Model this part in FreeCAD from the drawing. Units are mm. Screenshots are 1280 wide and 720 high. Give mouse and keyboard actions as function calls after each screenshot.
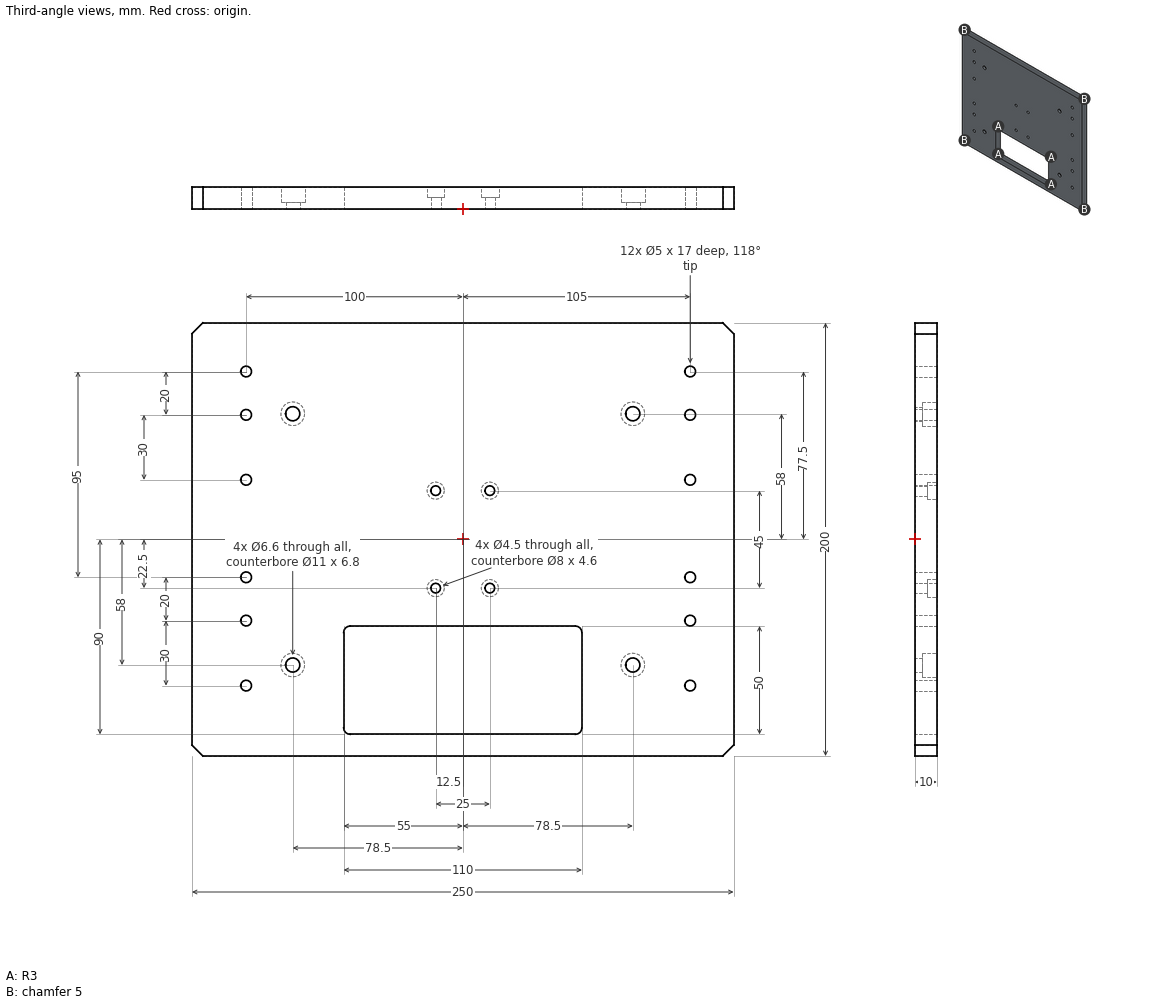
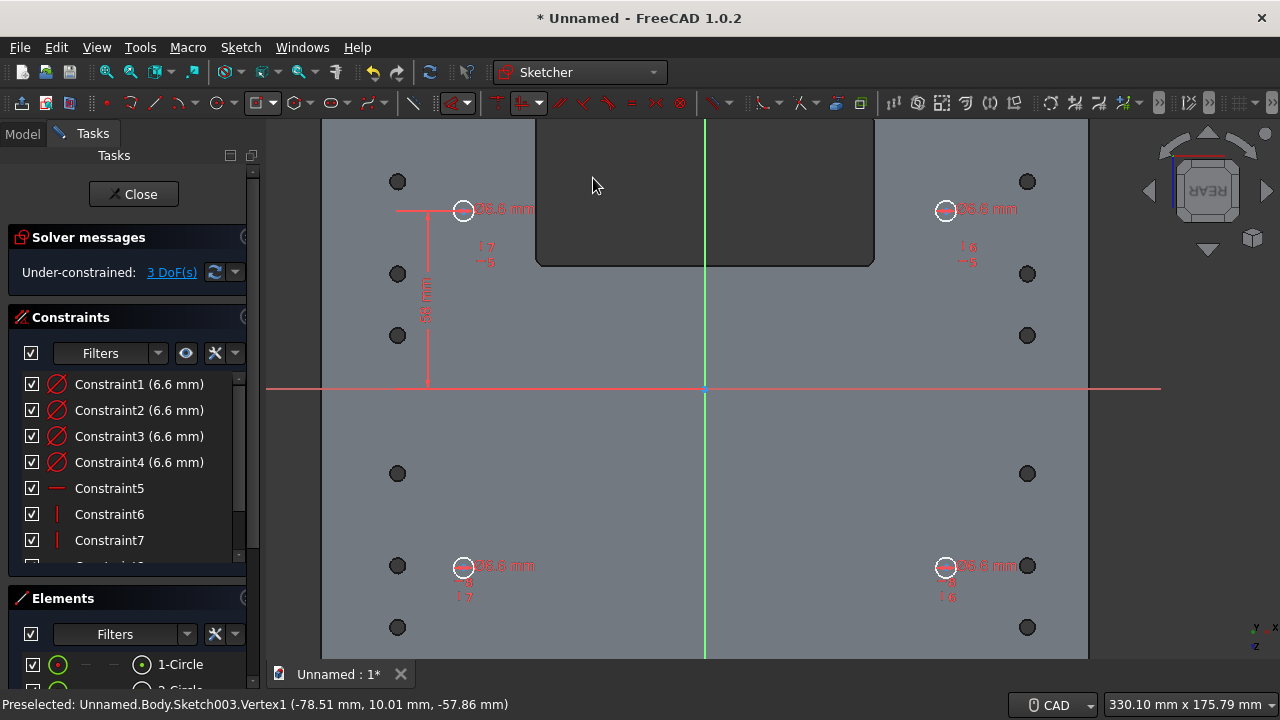
click(946, 568)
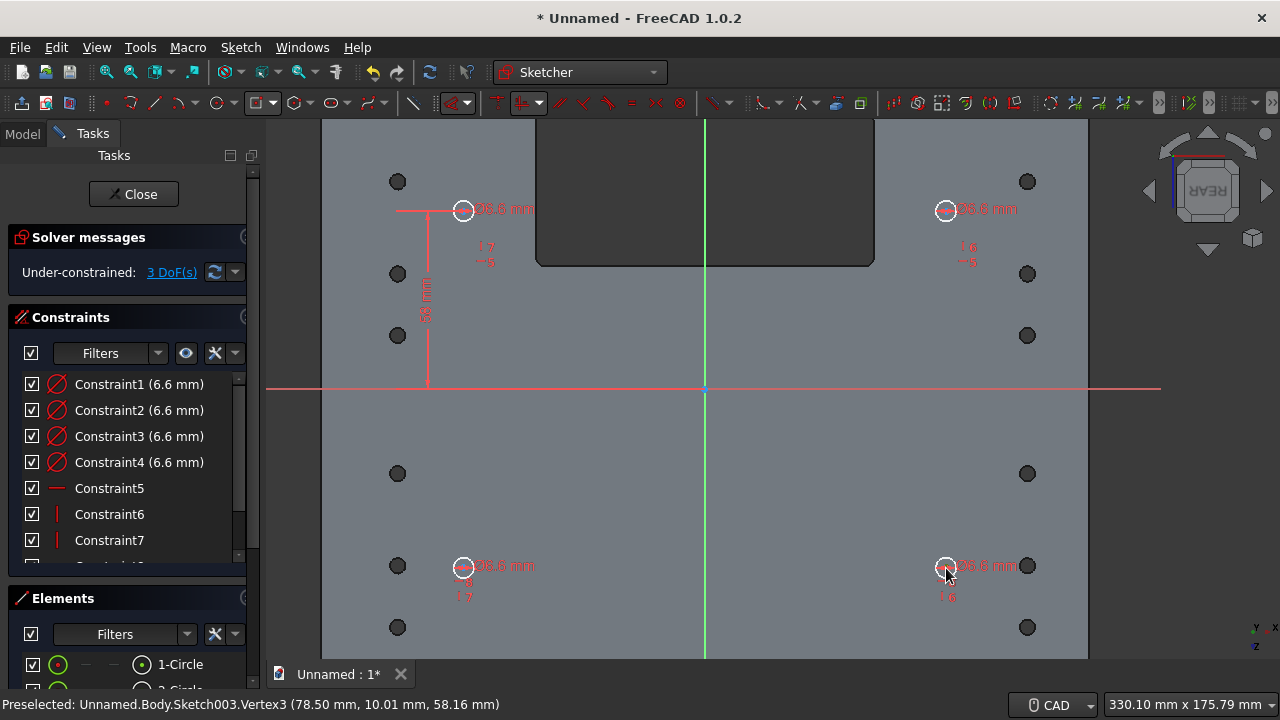
key(i)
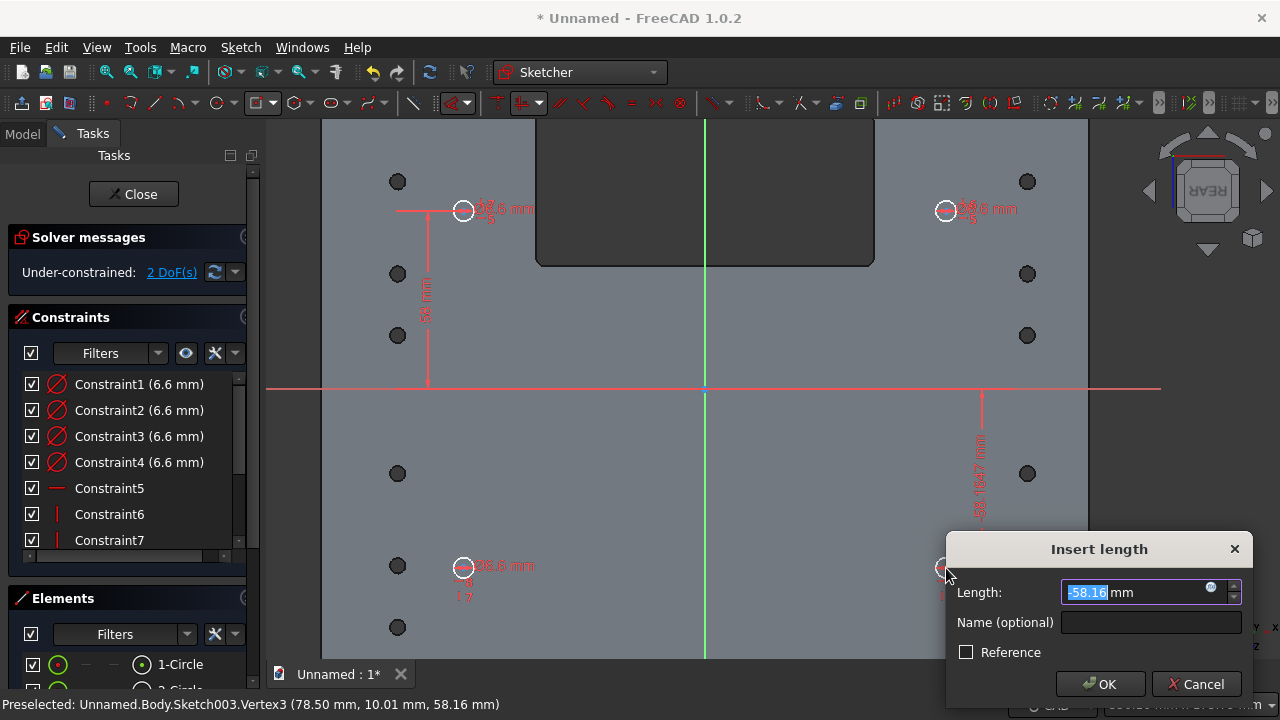
text(-58)
key(Return)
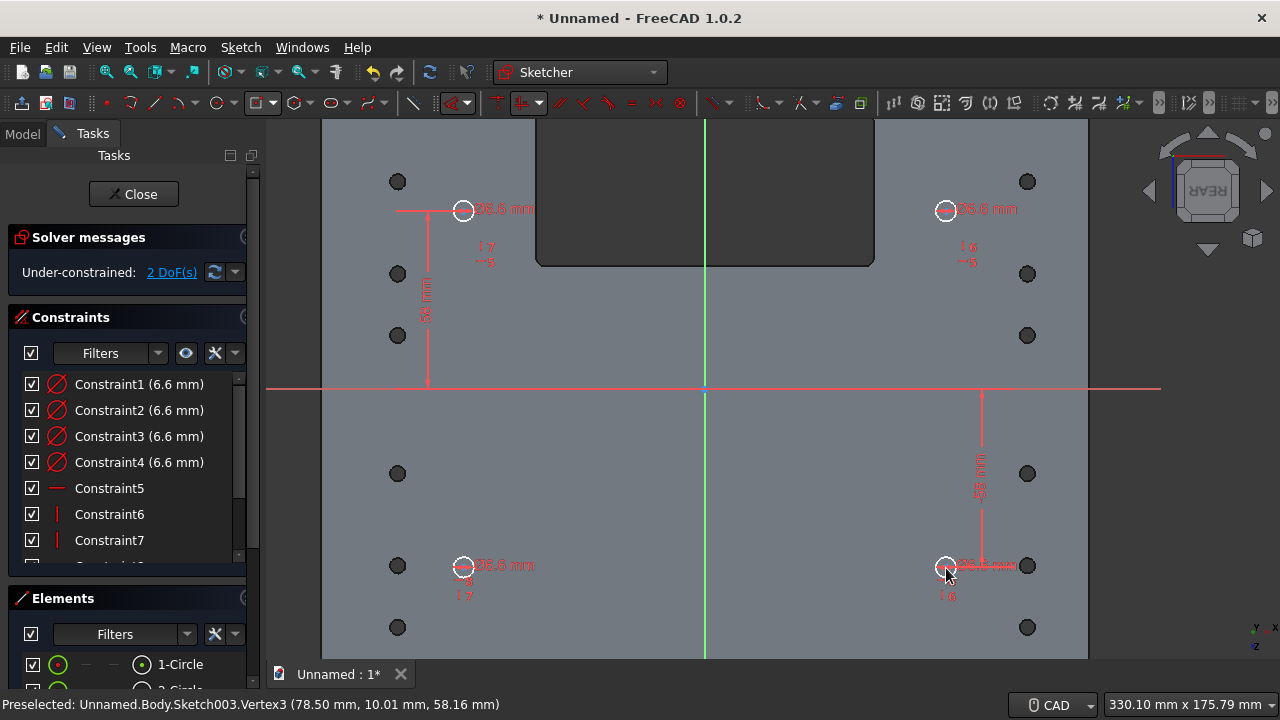
click(464, 211)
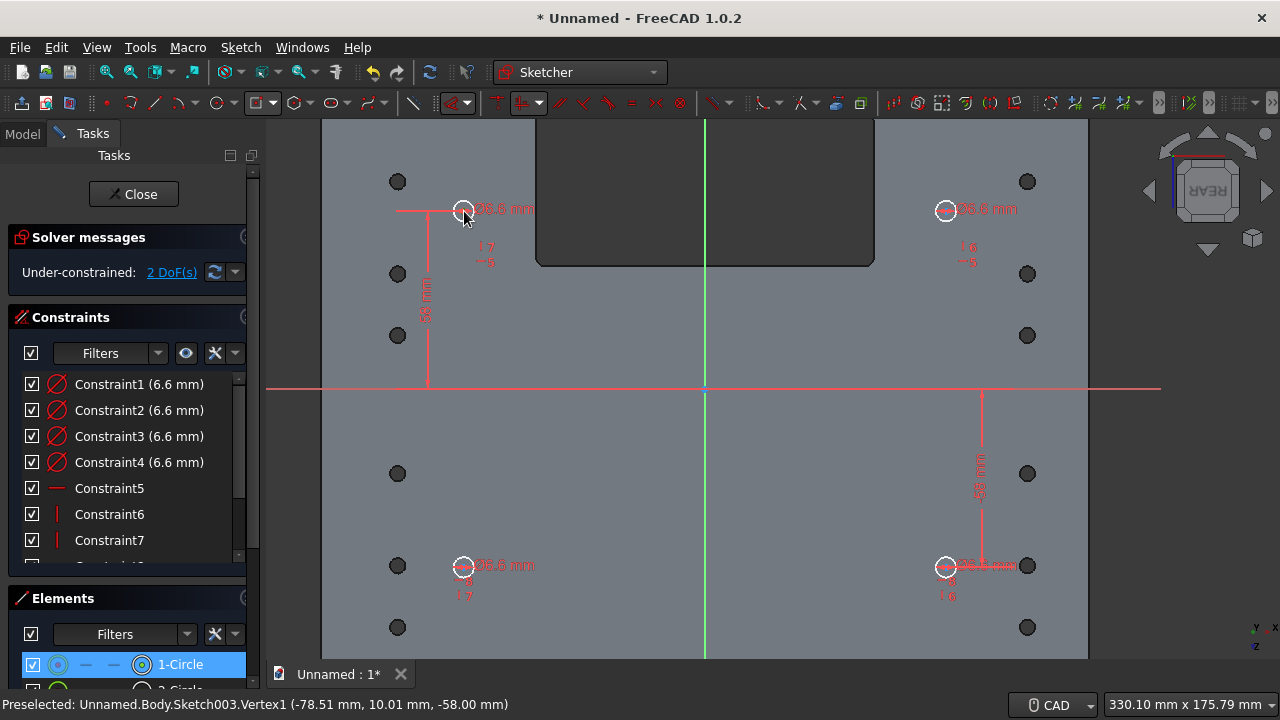
click(470, 104)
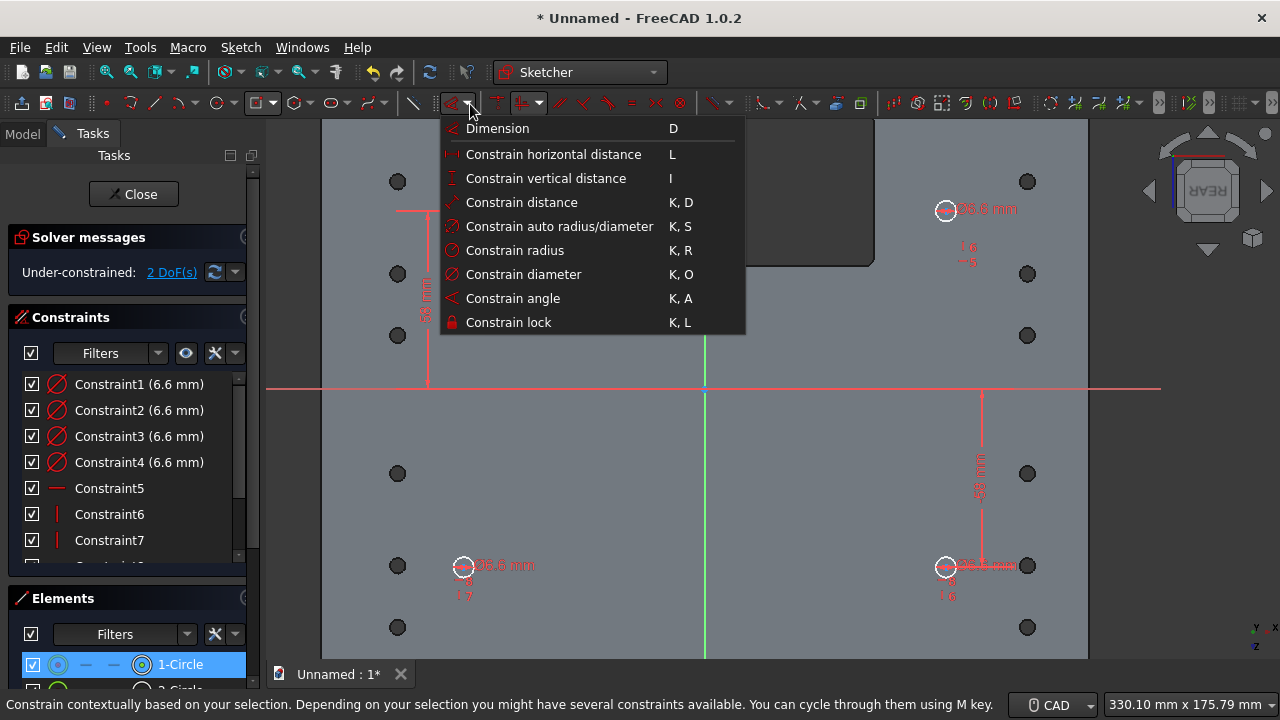
click(593, 154)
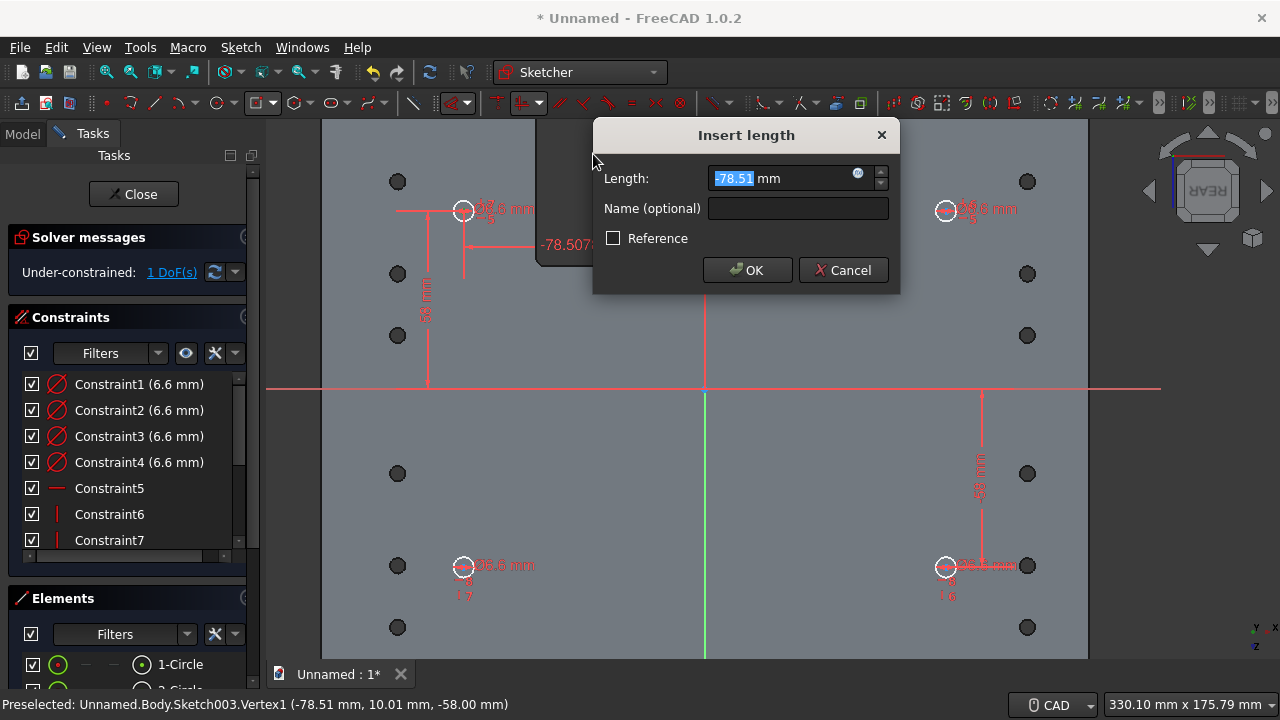
text(-78.5)
key(Return)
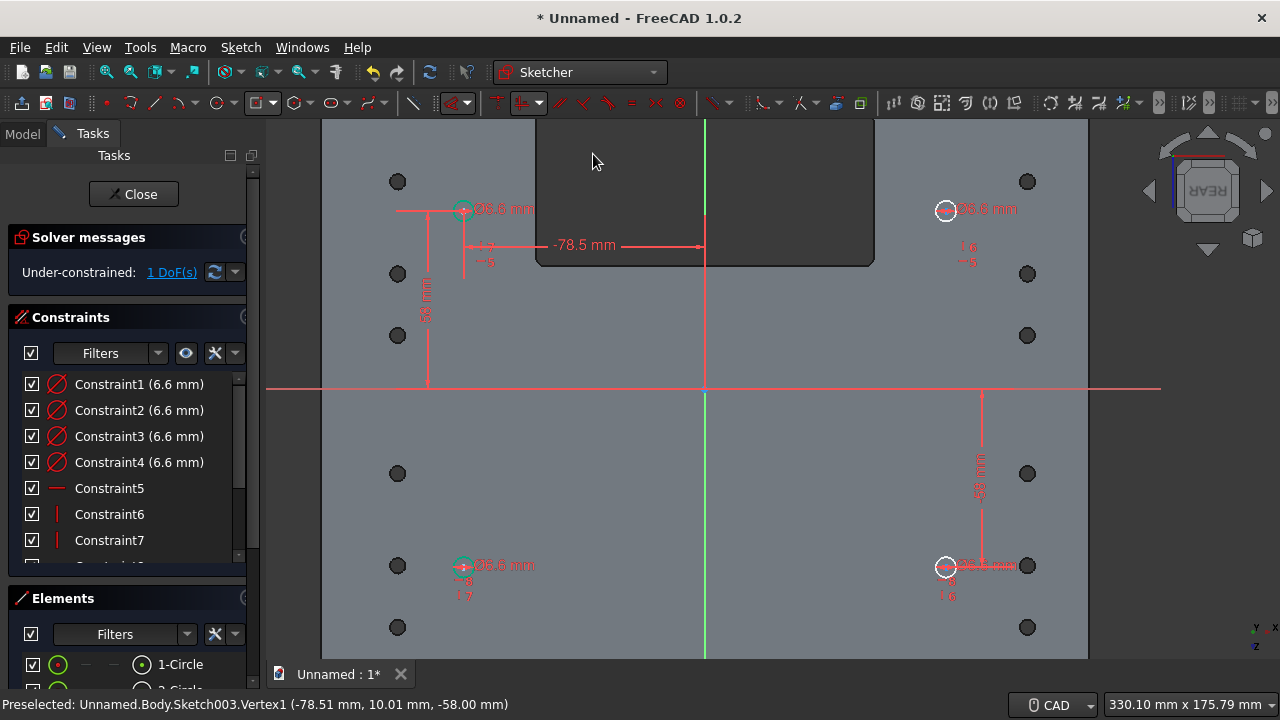
click(946, 211)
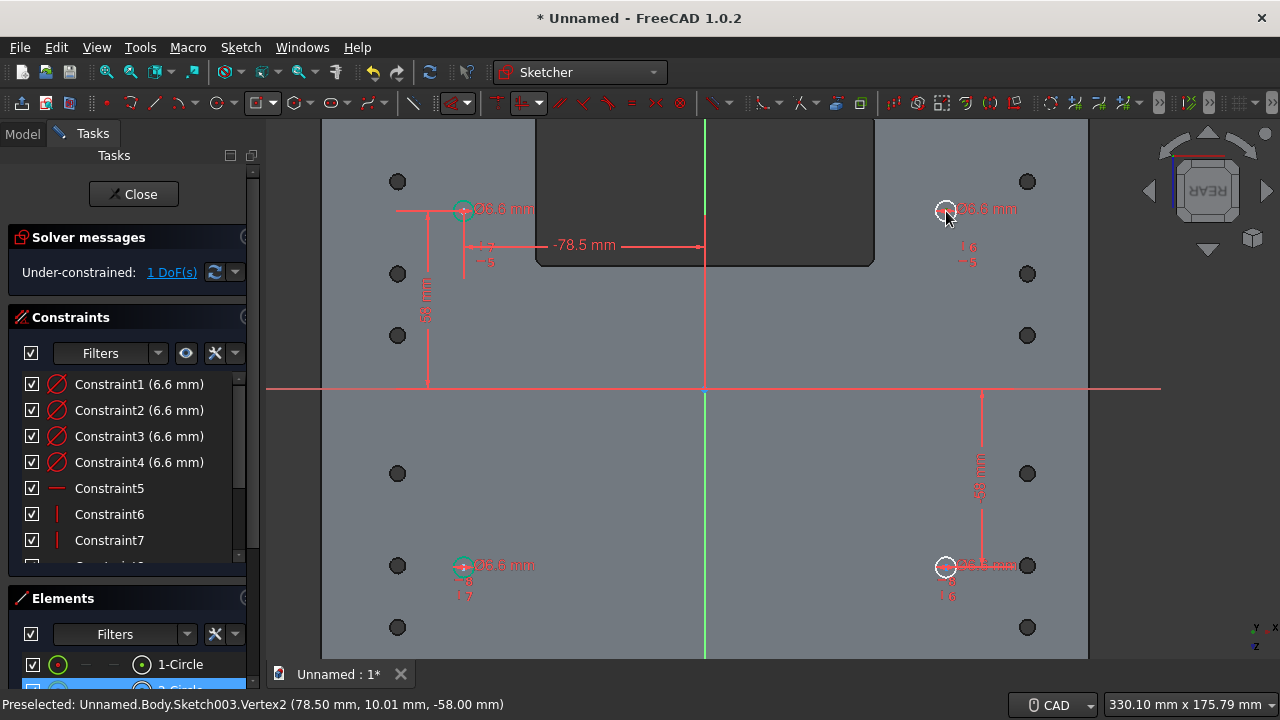
click(470, 104)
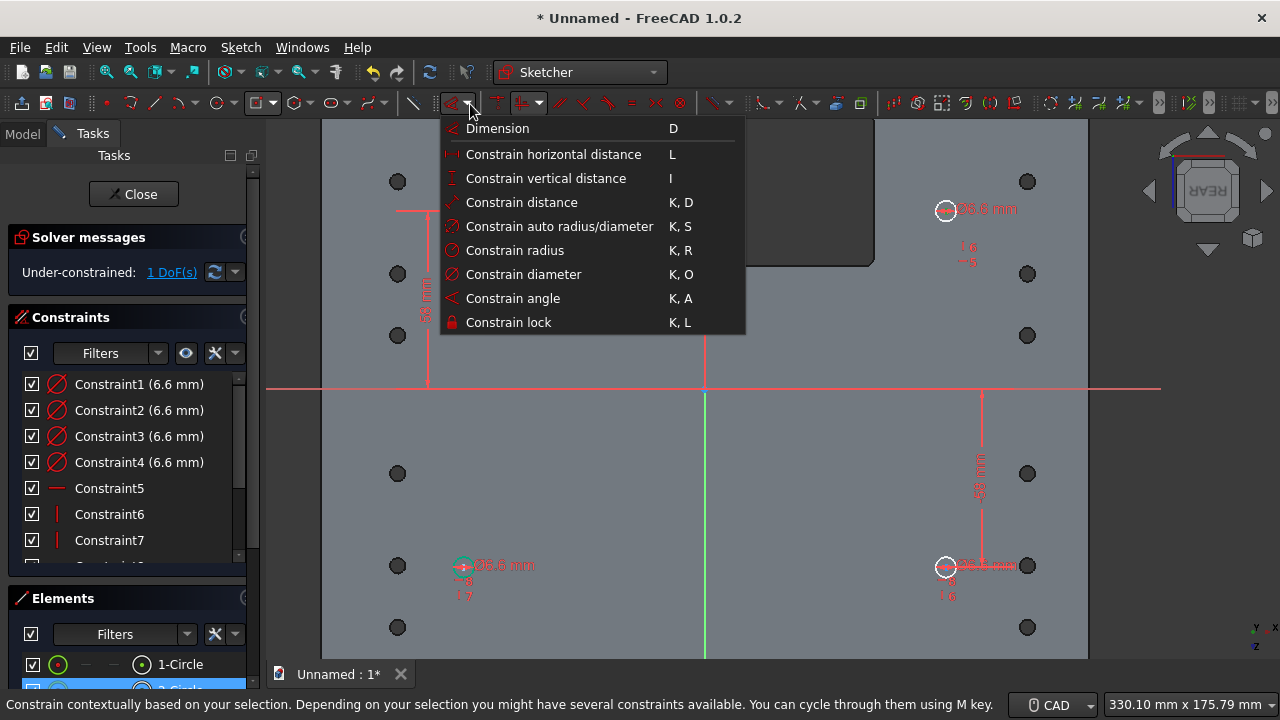
click(593, 154)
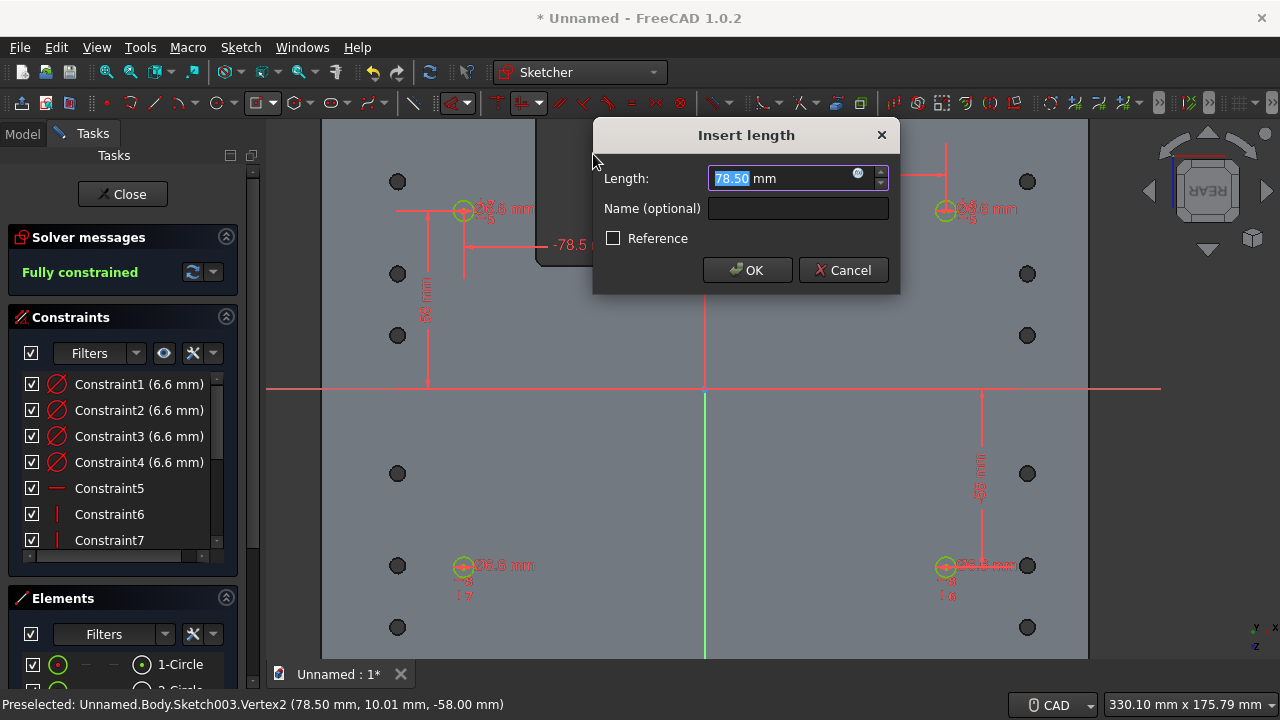
text(78.5)
key(Return)